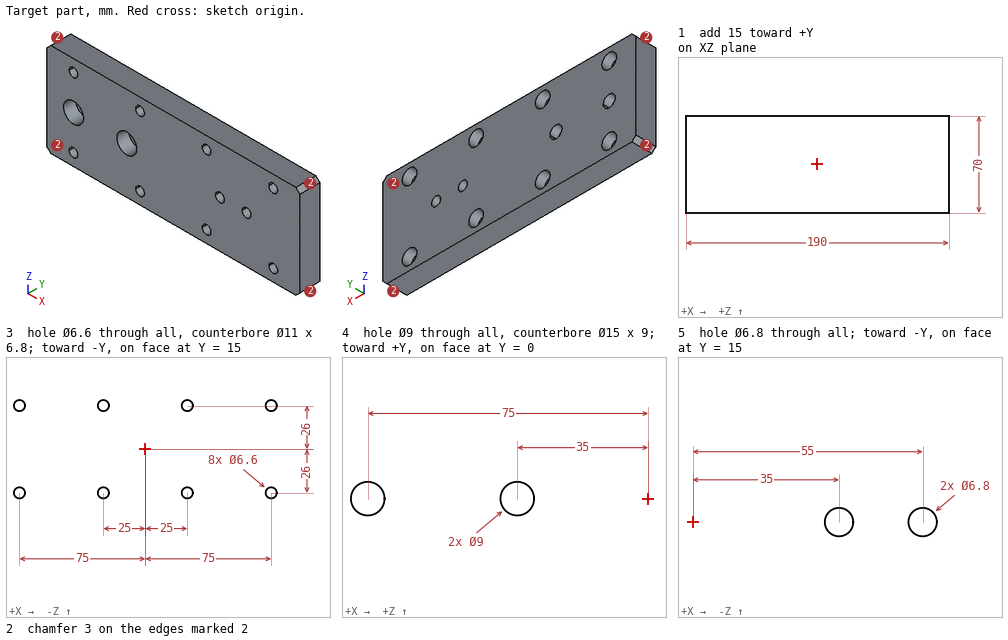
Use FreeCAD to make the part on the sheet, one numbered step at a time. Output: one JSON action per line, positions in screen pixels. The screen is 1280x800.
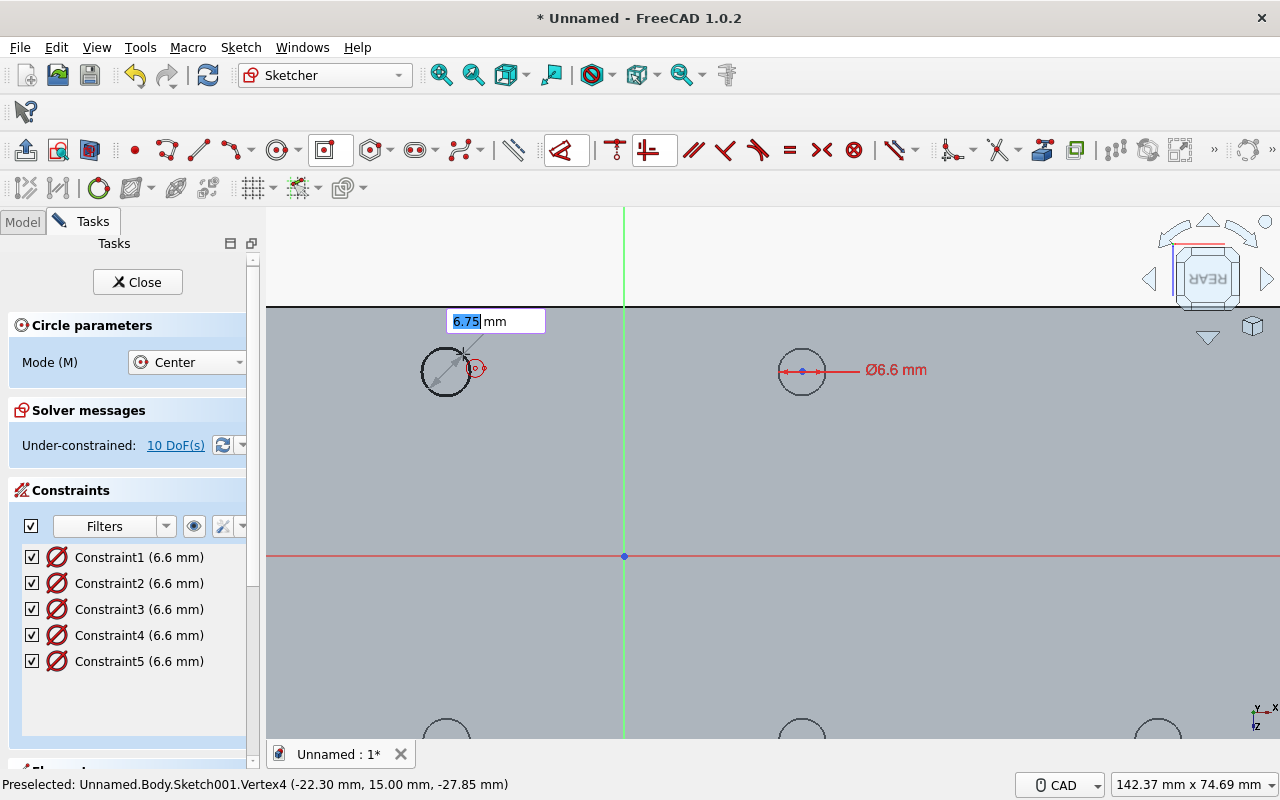
{"action": "type", "text": "6.6"}
{"action": "key", "text": "Return"}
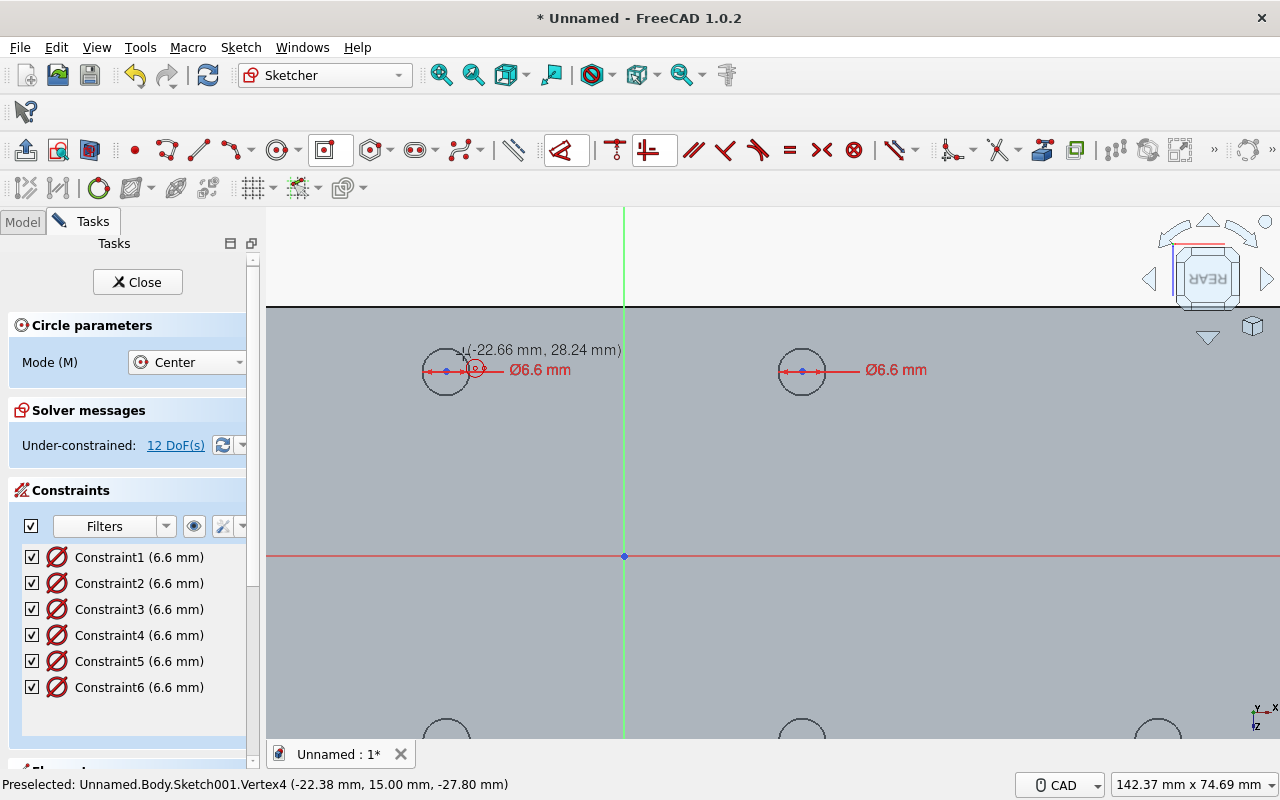
{"action": "scroll", "coordinate": [802, 372], "scroll_direction": "down", "scroll_amount": 3}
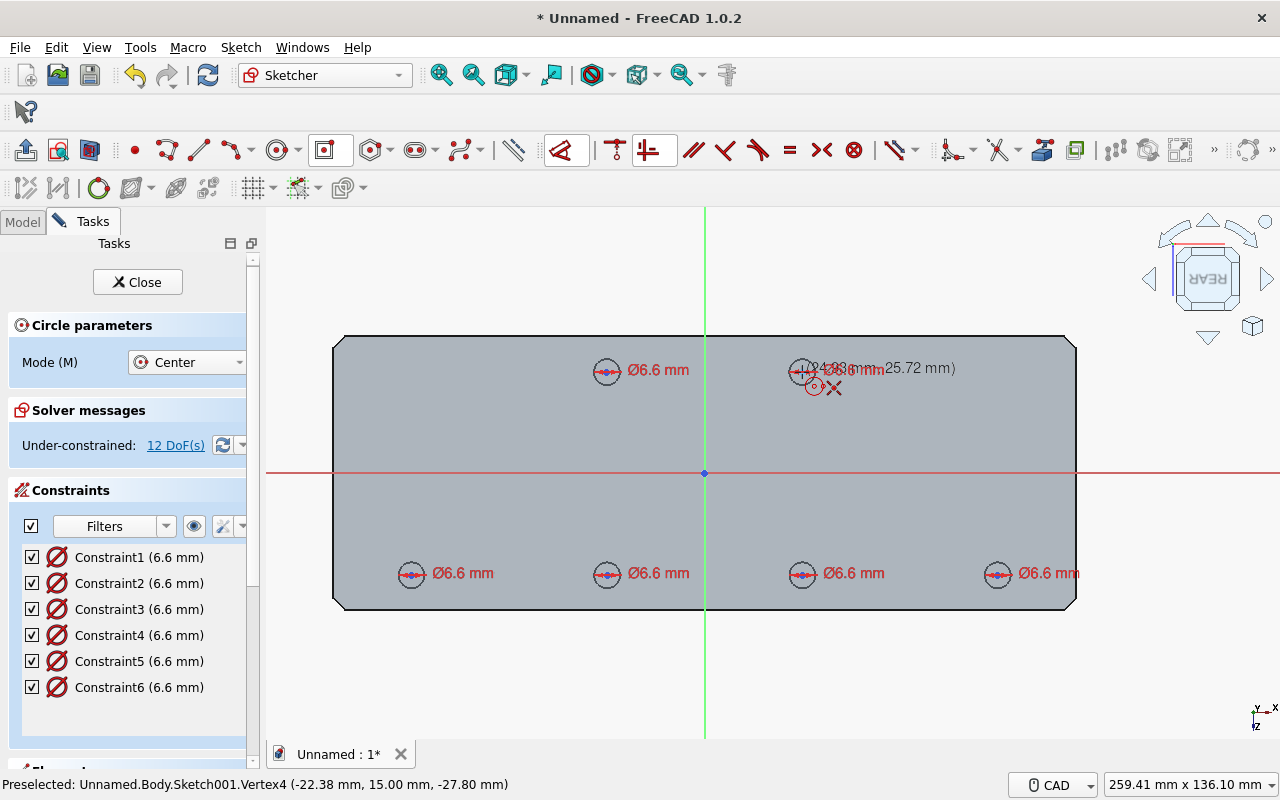
{"action": "scroll", "coordinate": [412, 372], "scroll_direction": "up", "scroll_amount": 3}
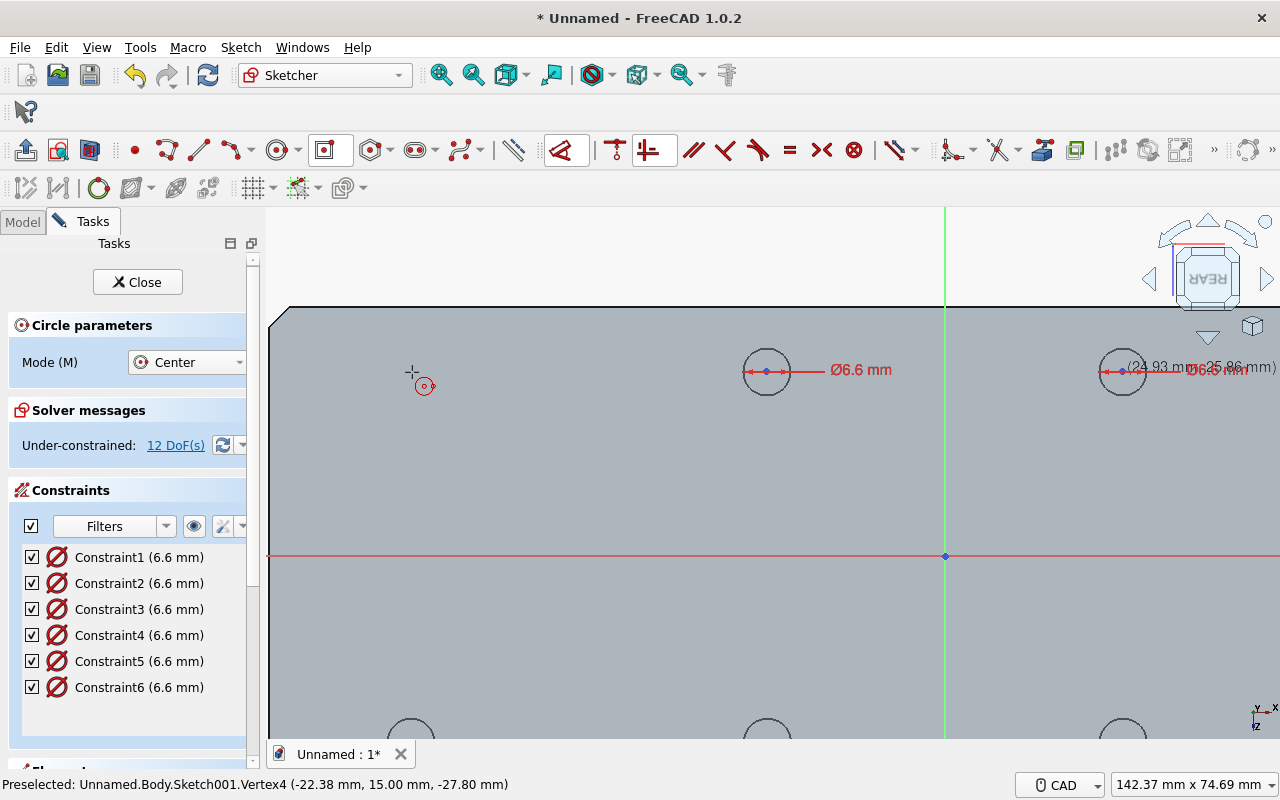
{"action": "left_click", "coordinate": [411, 371]}
{"action": "mouse_move", "coordinate": [428, 354]}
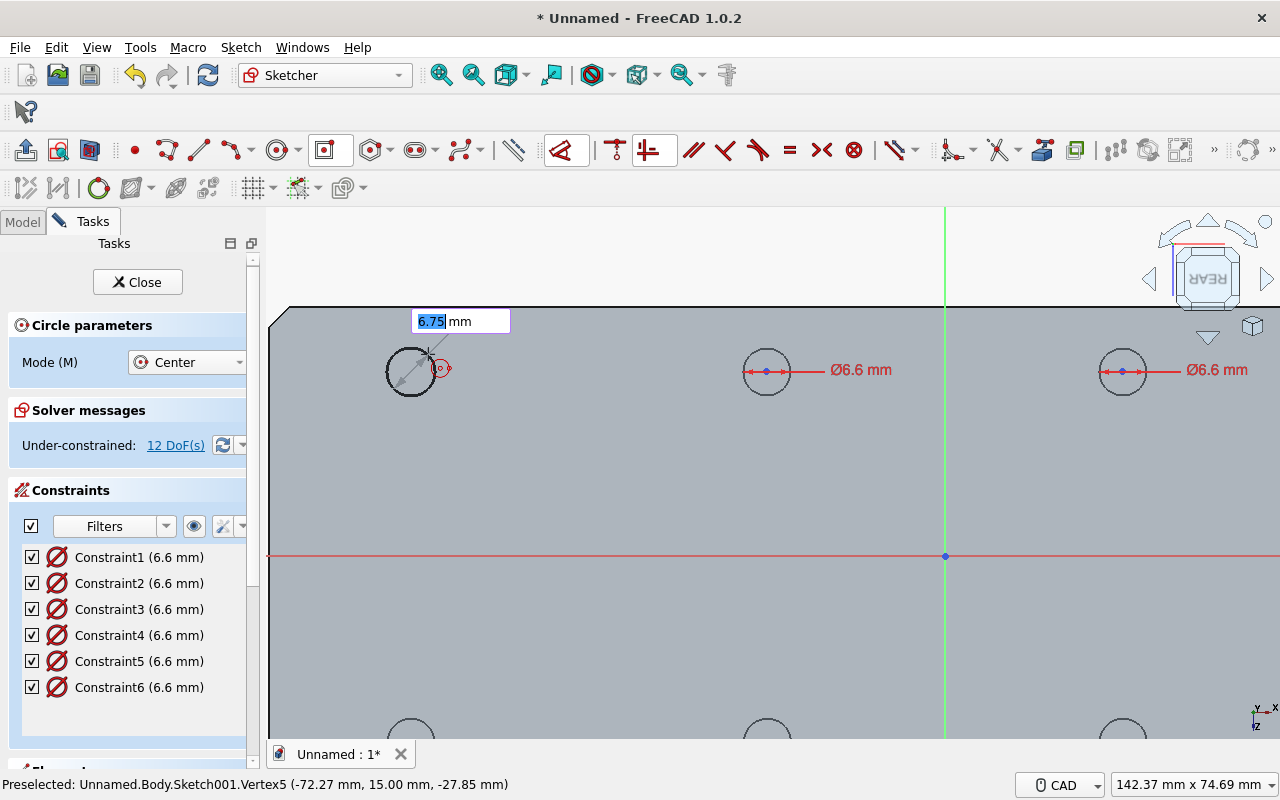
{"action": "type", "text": "6.6"}
{"action": "key", "text": "Return"}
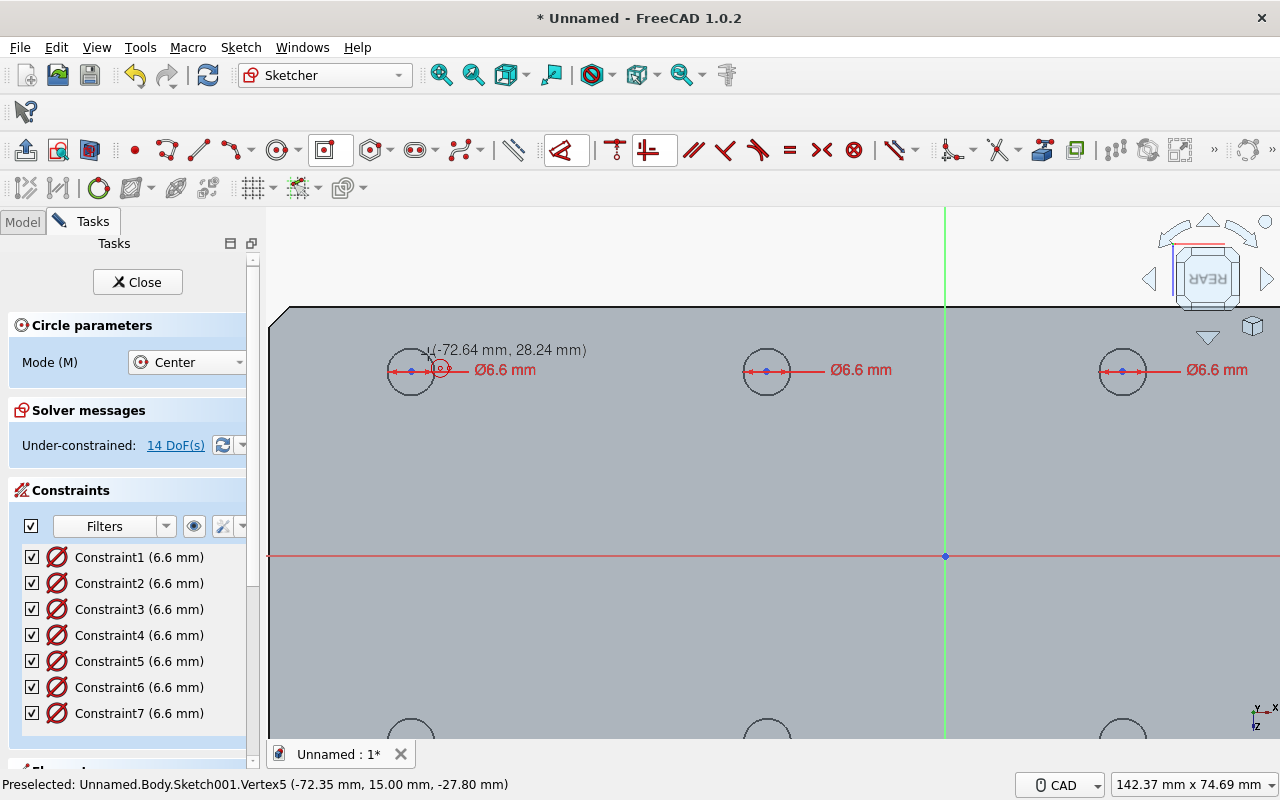
{"action": "scroll", "coordinate": [412, 372], "scroll_direction": "down", "scroll_amount": 3}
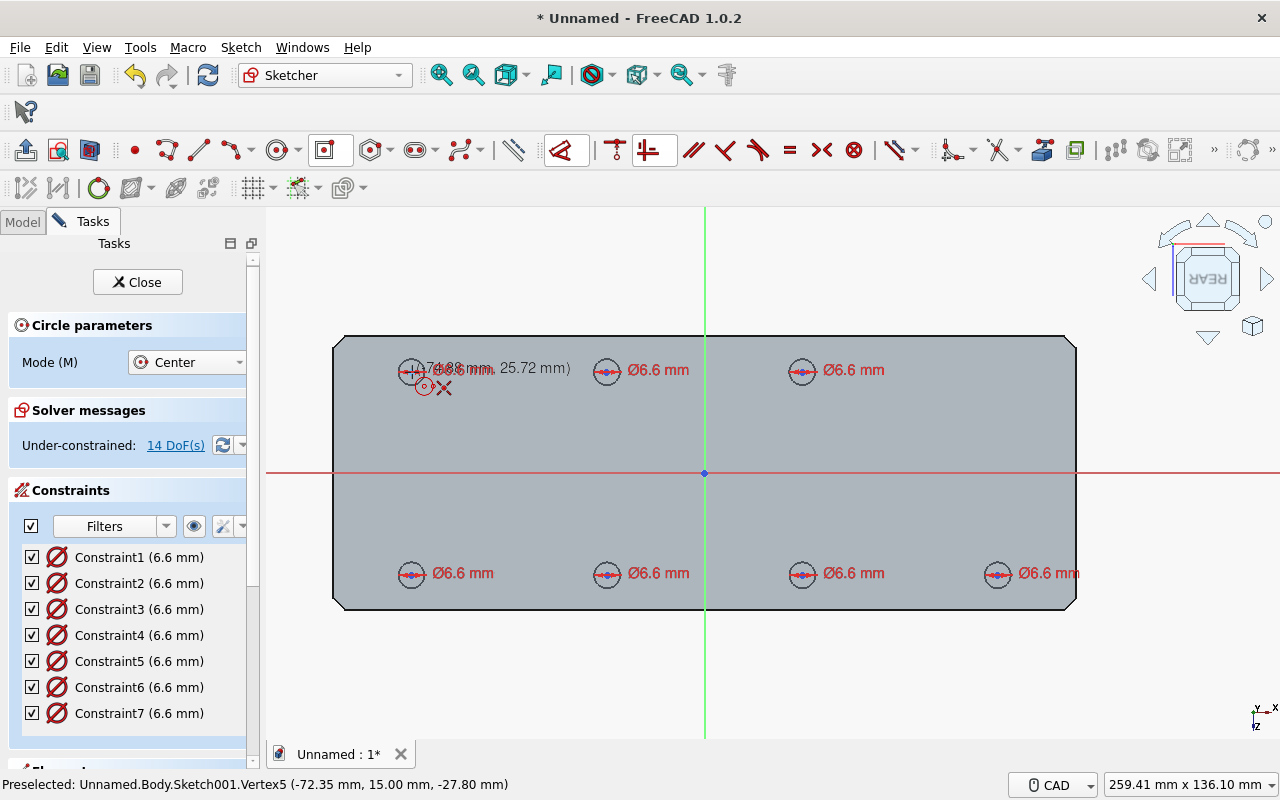
{"action": "scroll", "coordinate": [998, 372], "scroll_direction": "up", "scroll_amount": 3}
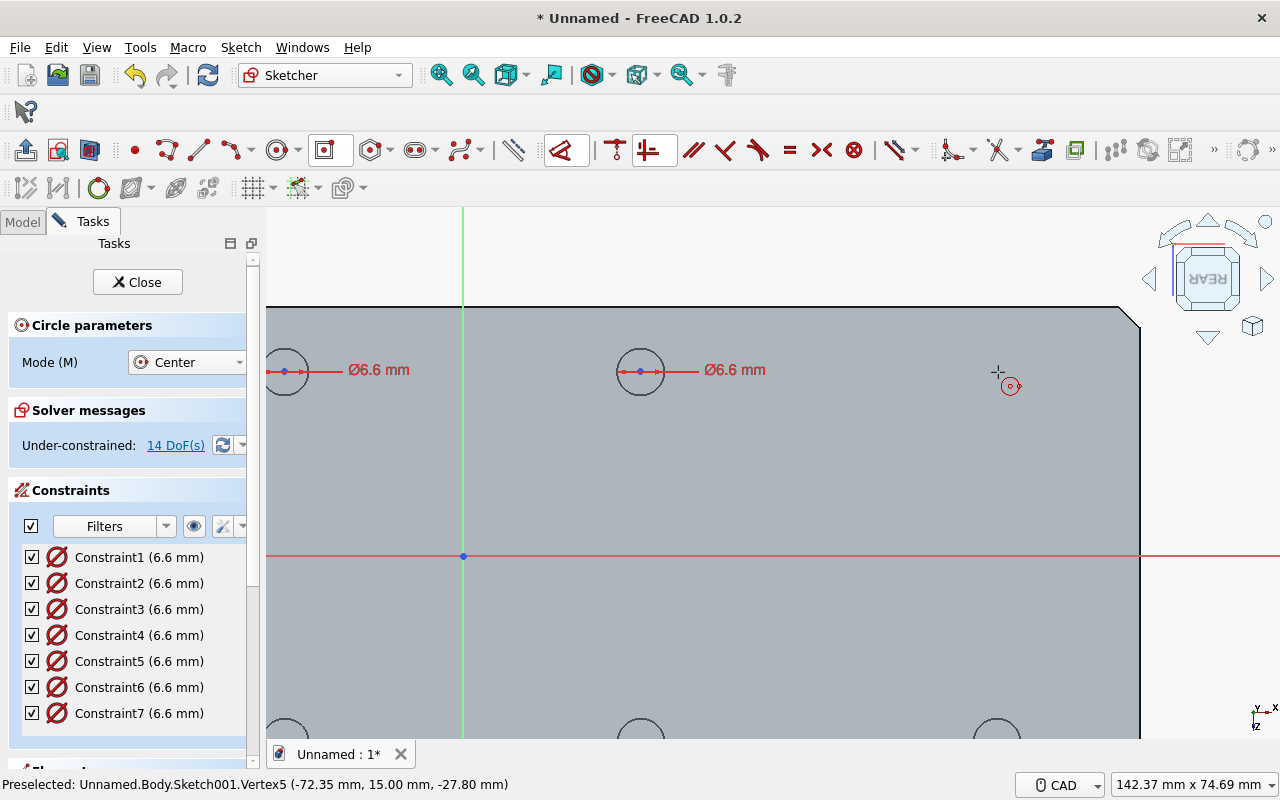
{"action": "left_click", "coordinate": [997, 371]}
{"action": "mouse_move", "coordinate": [1014, 354]}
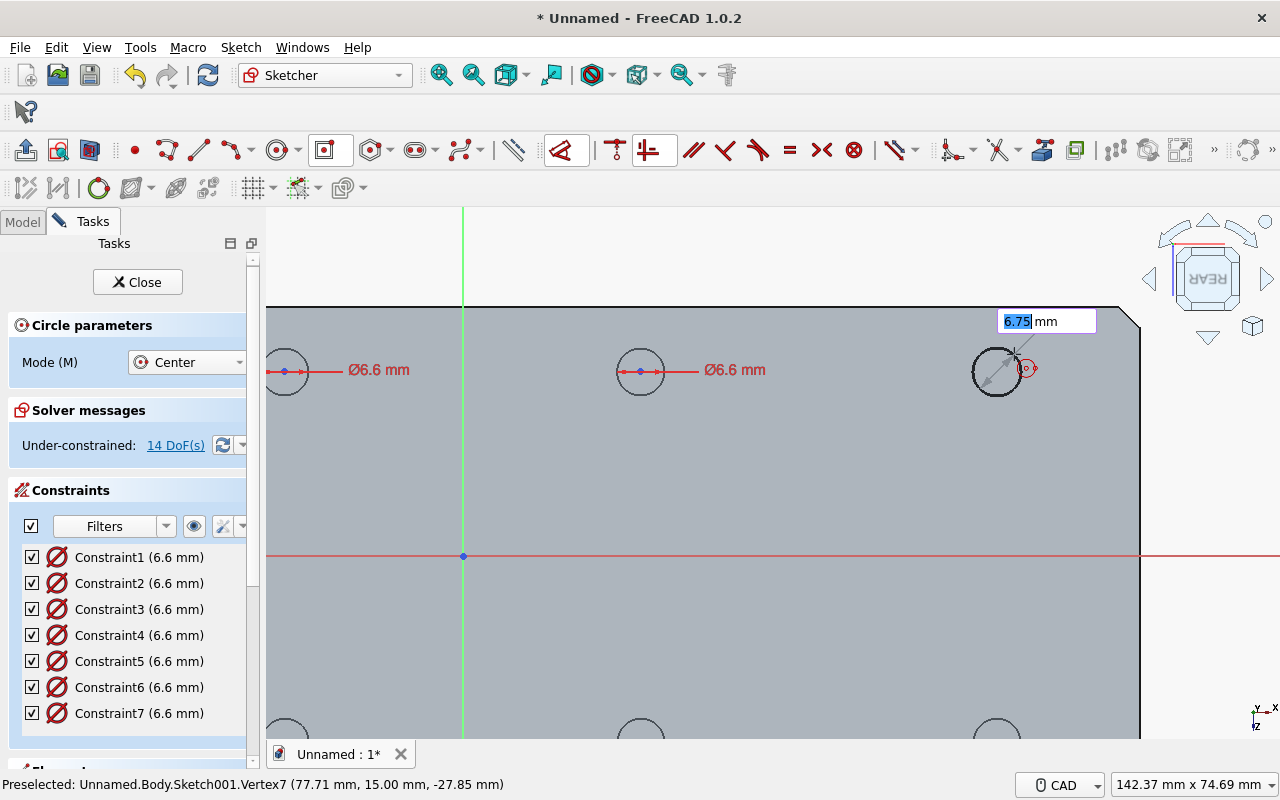
{"action": "type", "text": "6.6"}
{"action": "key", "text": "Return"}
{"action": "key", "text": "Escape"}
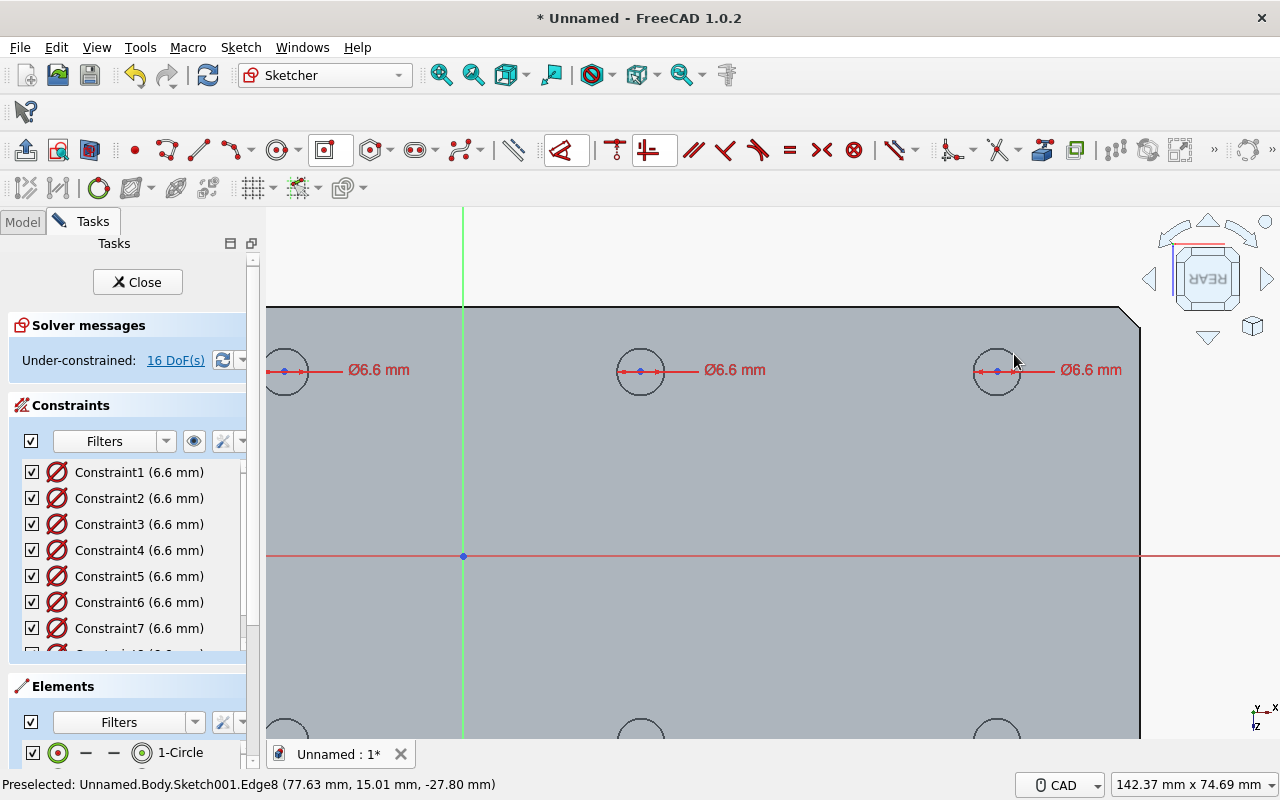
{"action": "scroll", "coordinate": [998, 372], "scroll_direction": "down", "scroll_amount": 3}